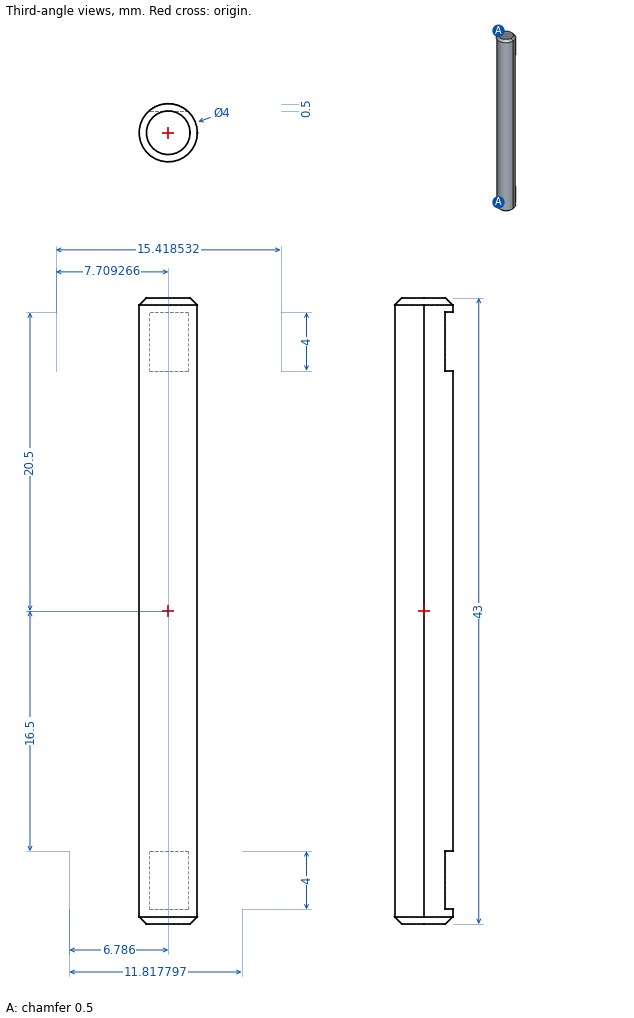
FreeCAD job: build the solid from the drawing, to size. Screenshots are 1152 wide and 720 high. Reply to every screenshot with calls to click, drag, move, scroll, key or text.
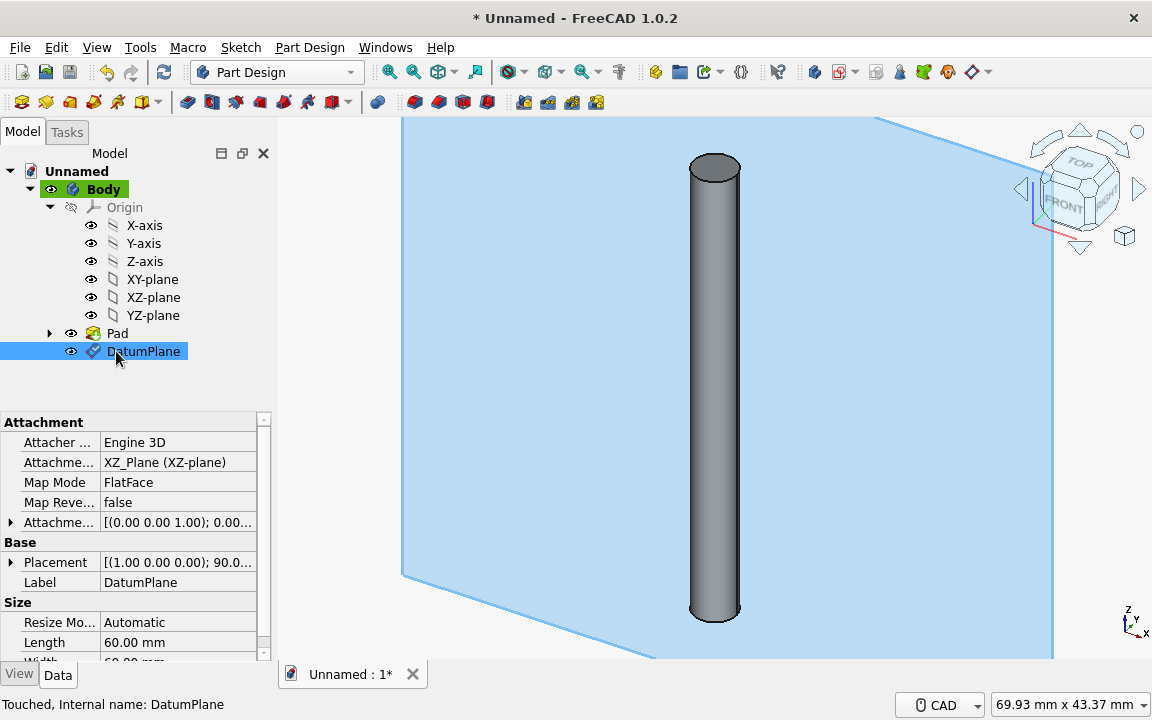
click(840, 72)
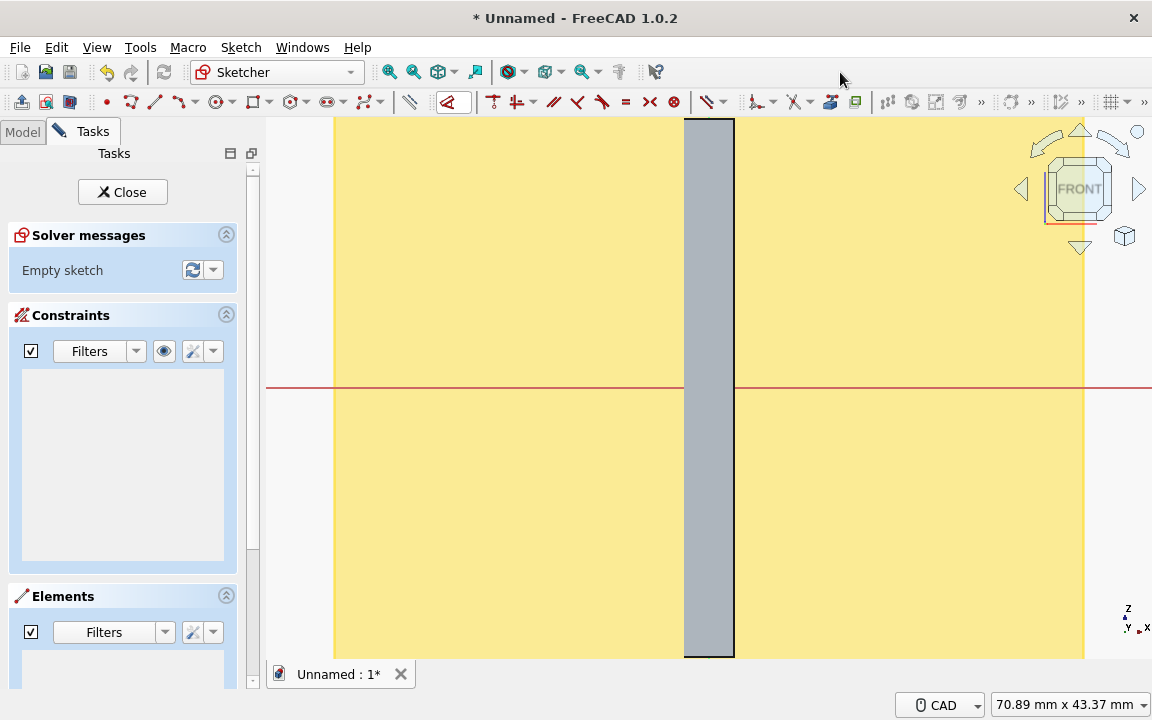
click(70, 102)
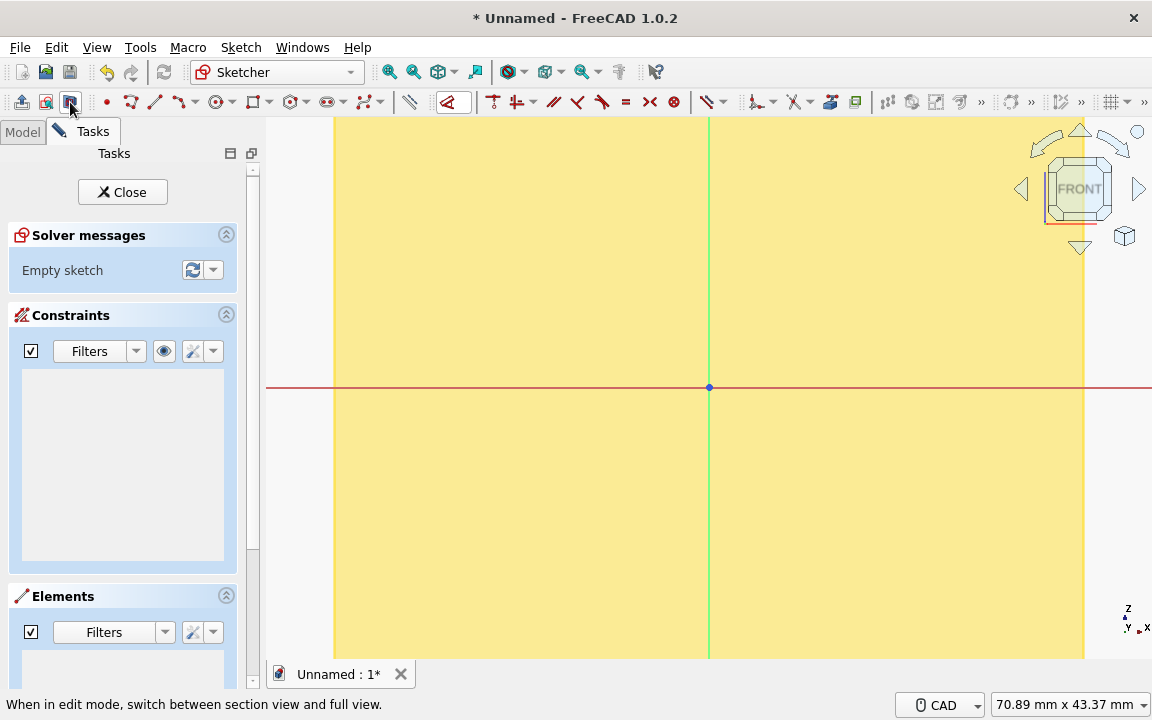
scroll(501, 388, down, 2)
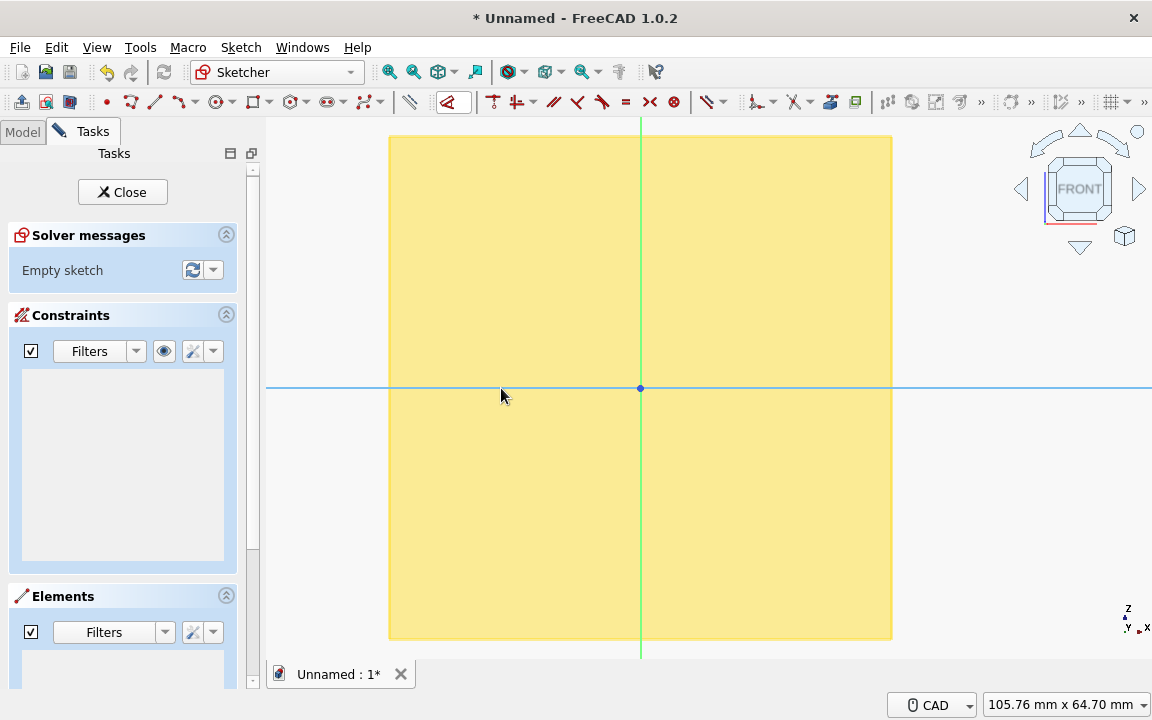
click(254, 102)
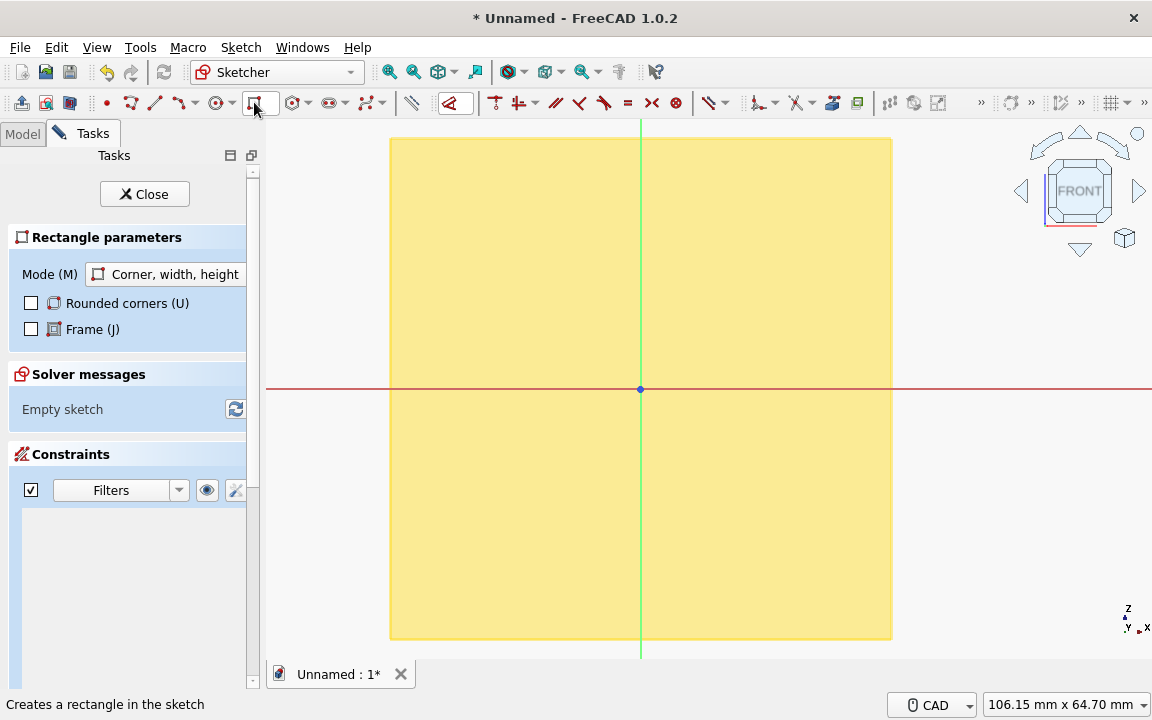
click(576, 218)
move(705, 251)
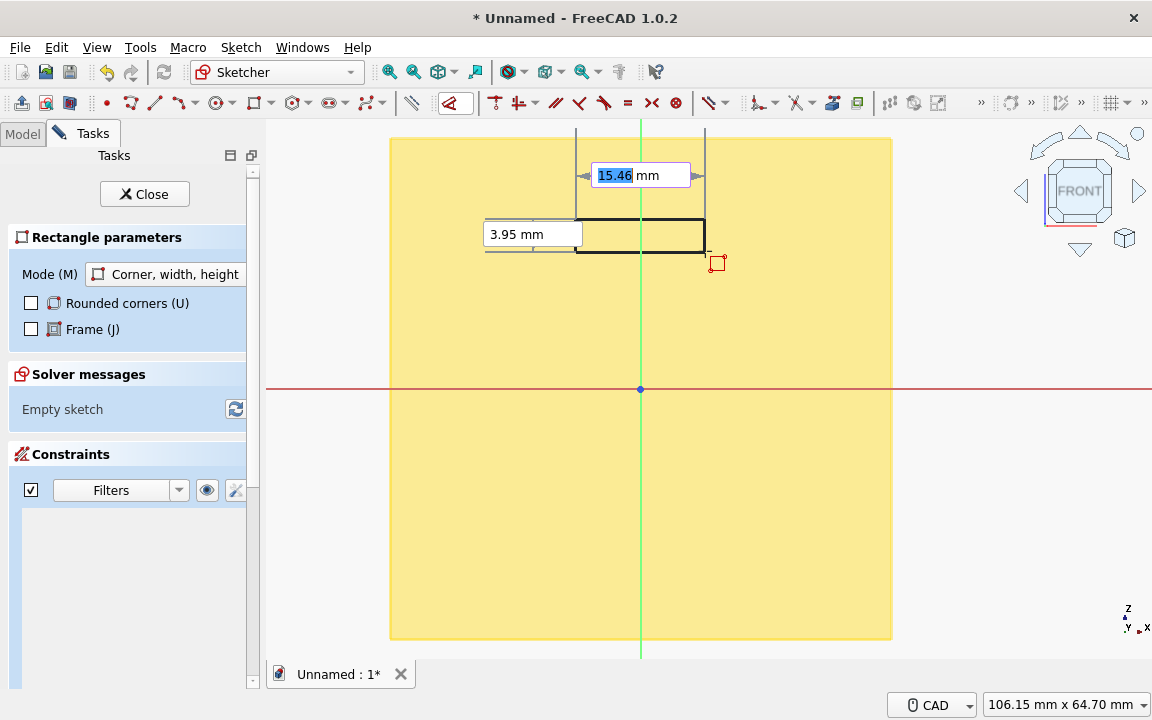
text(15.418532)
key(Tab)
text(4)
key(Return)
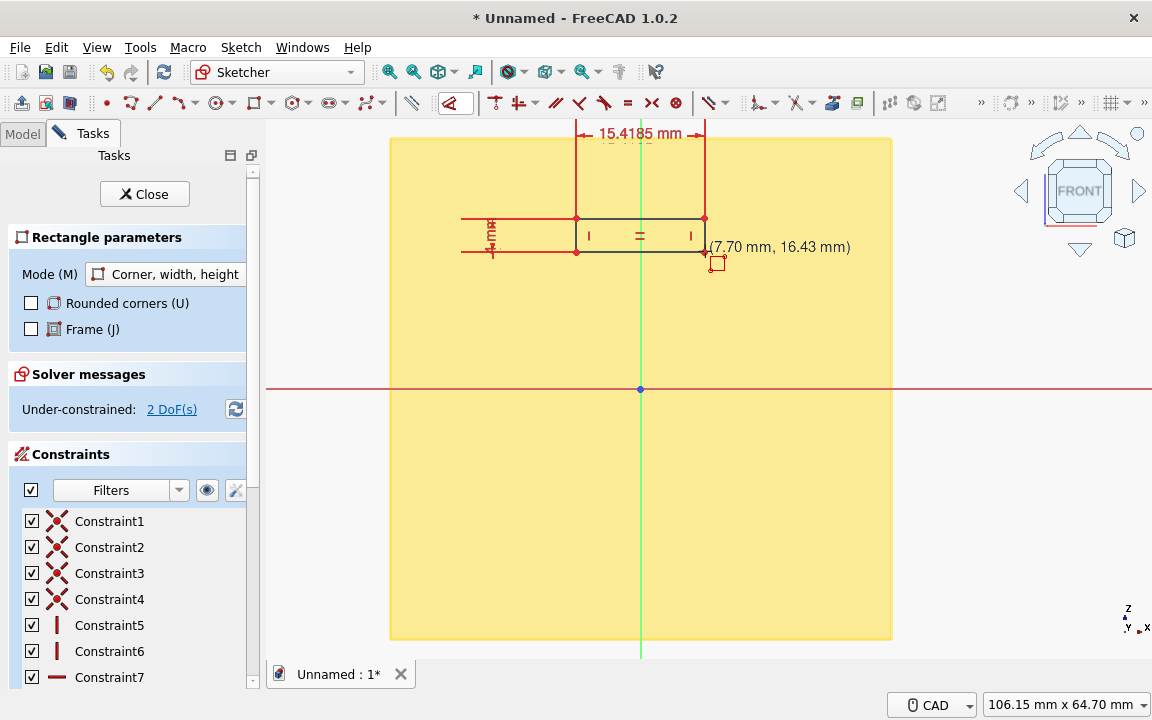
click(584, 527)
move(683, 560)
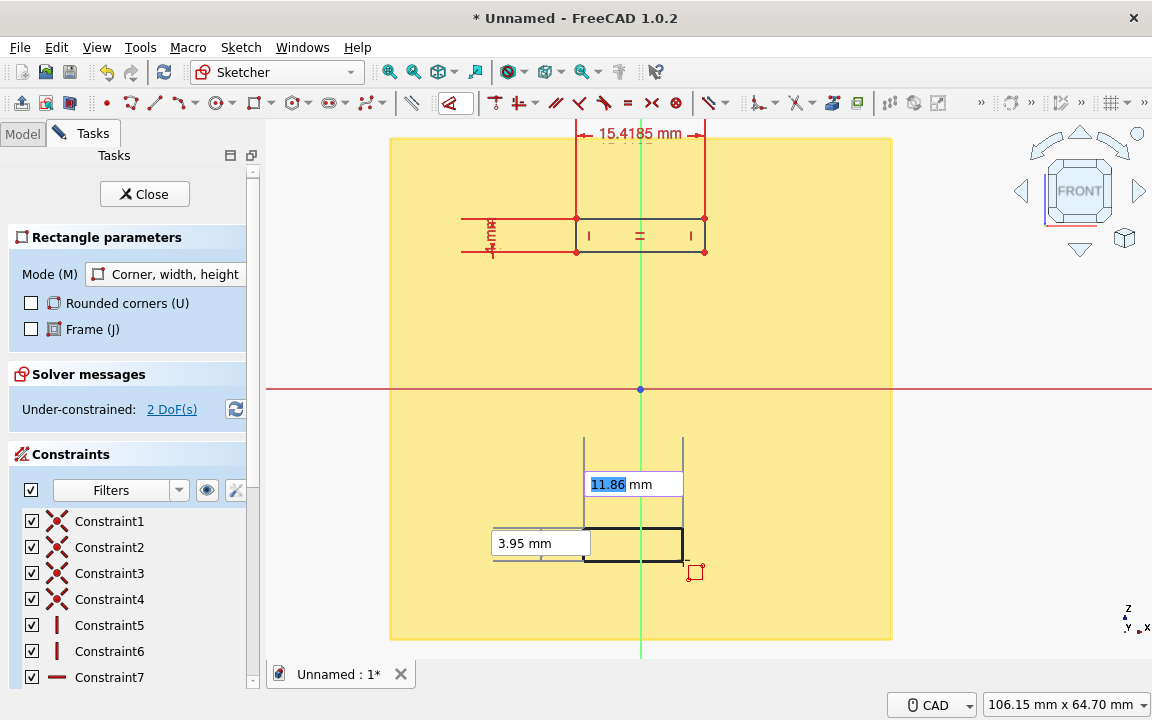
text(11.817797)
key(Tab)
text(4)
key(Return)
key(Escape)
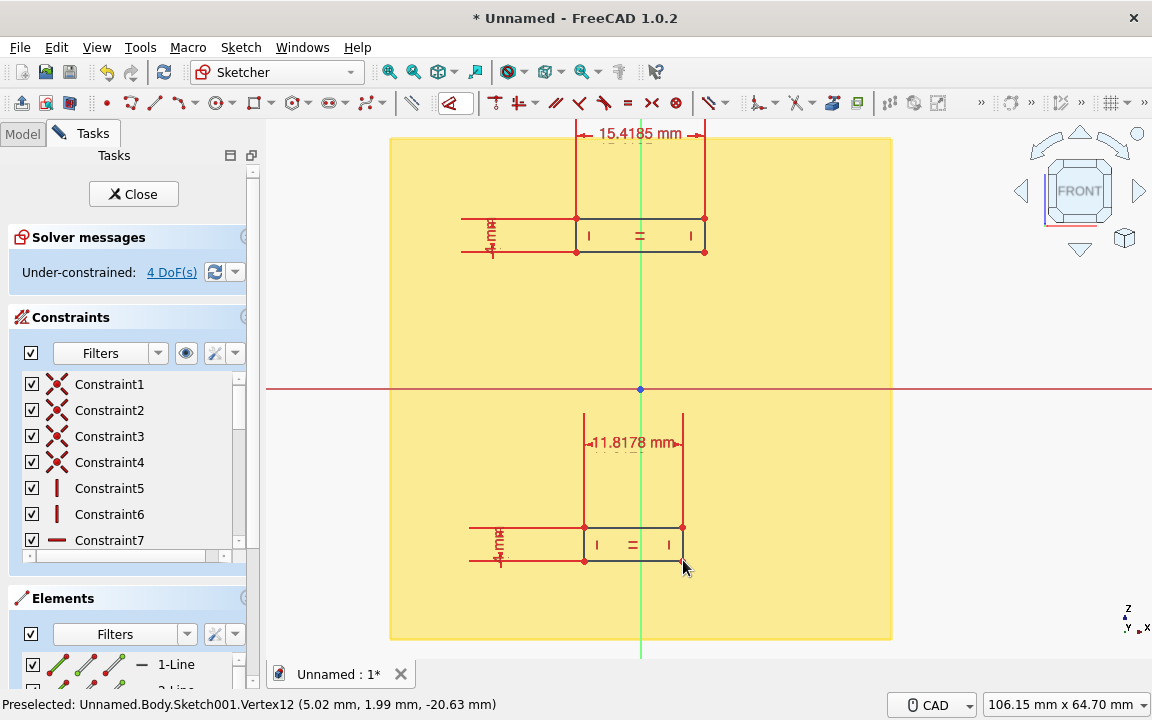
click(576, 219)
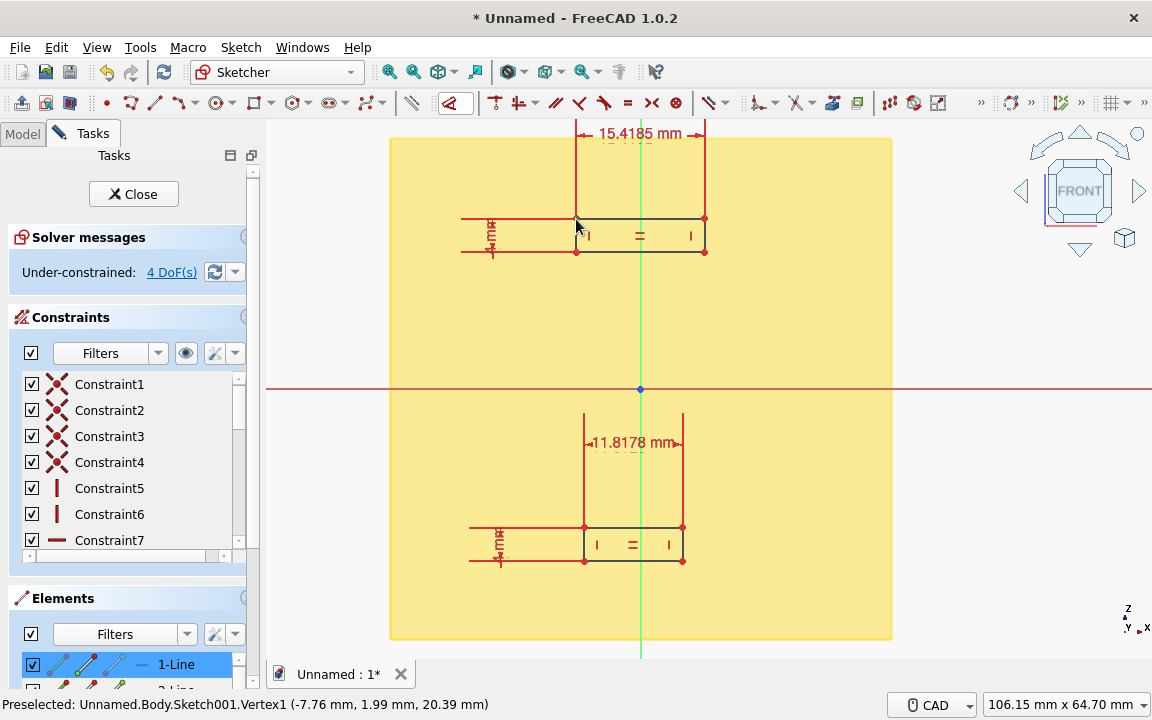
key(i)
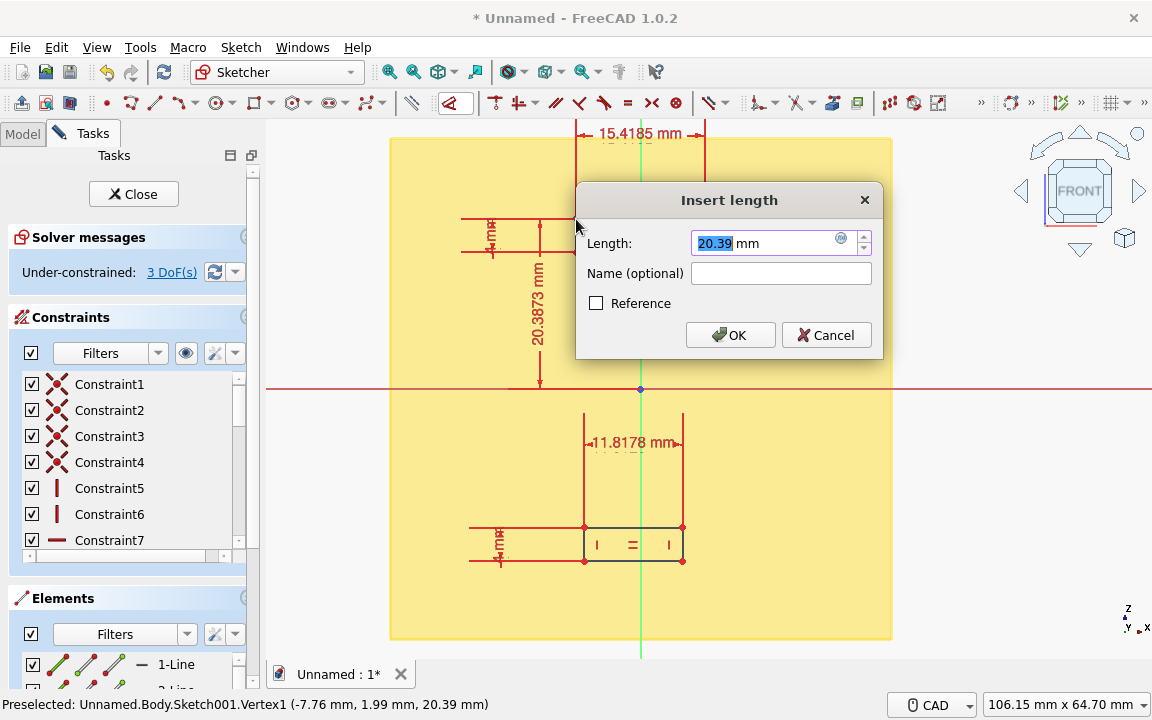
text(20.5)
key(Return)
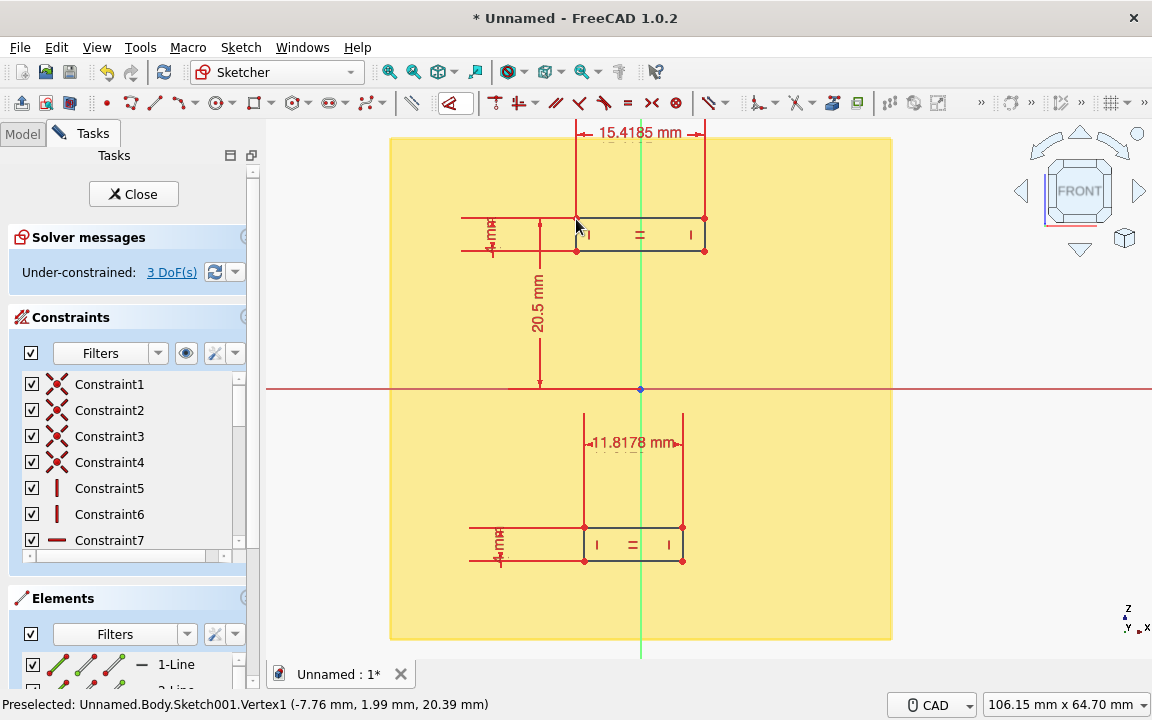
click(584, 528)